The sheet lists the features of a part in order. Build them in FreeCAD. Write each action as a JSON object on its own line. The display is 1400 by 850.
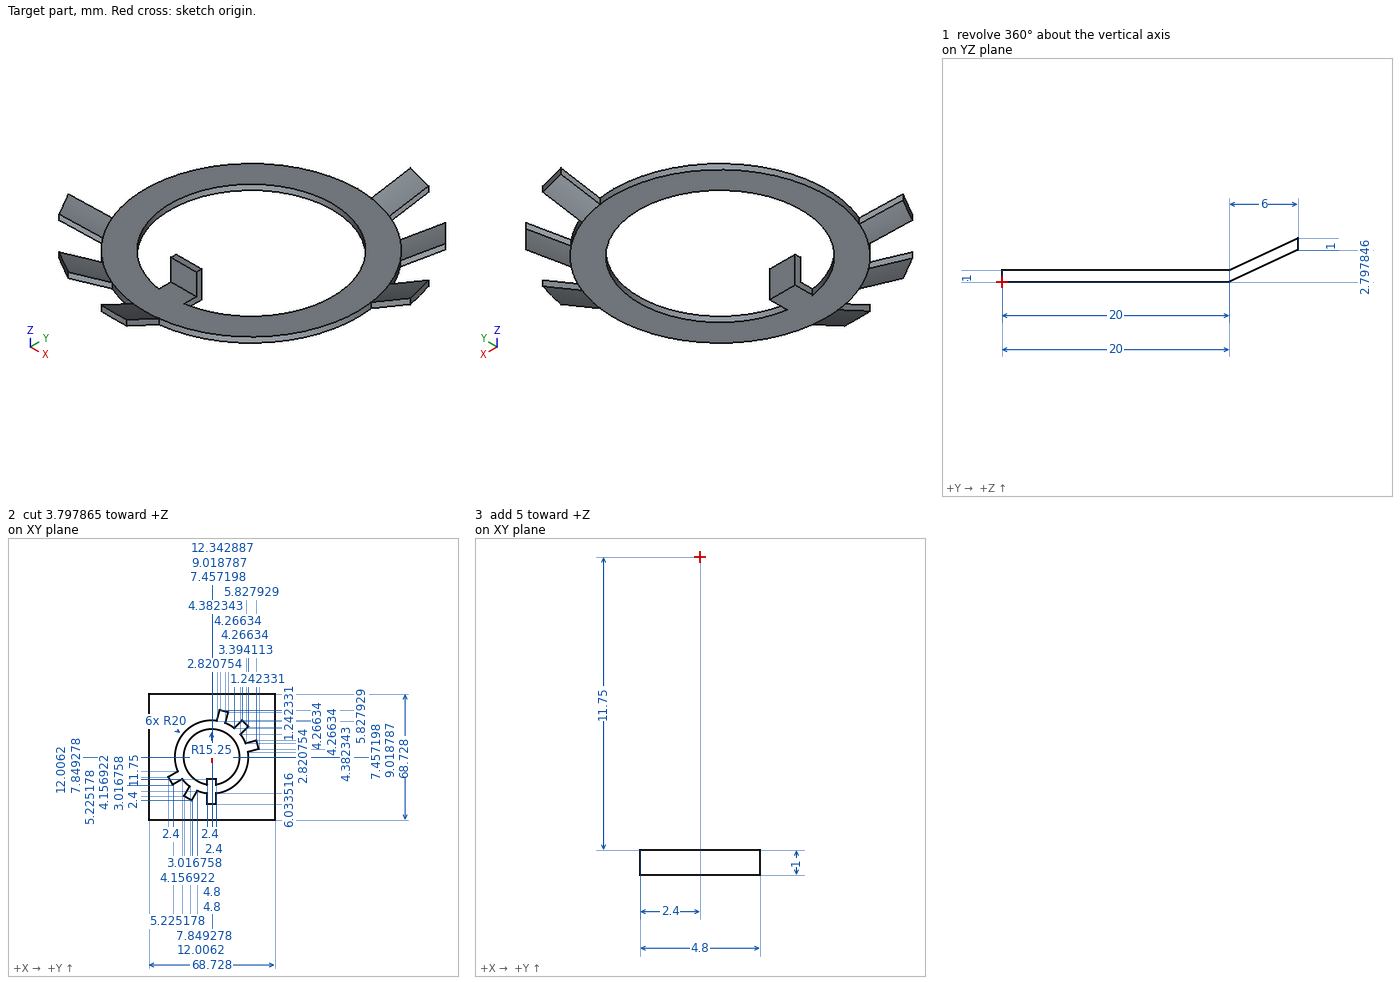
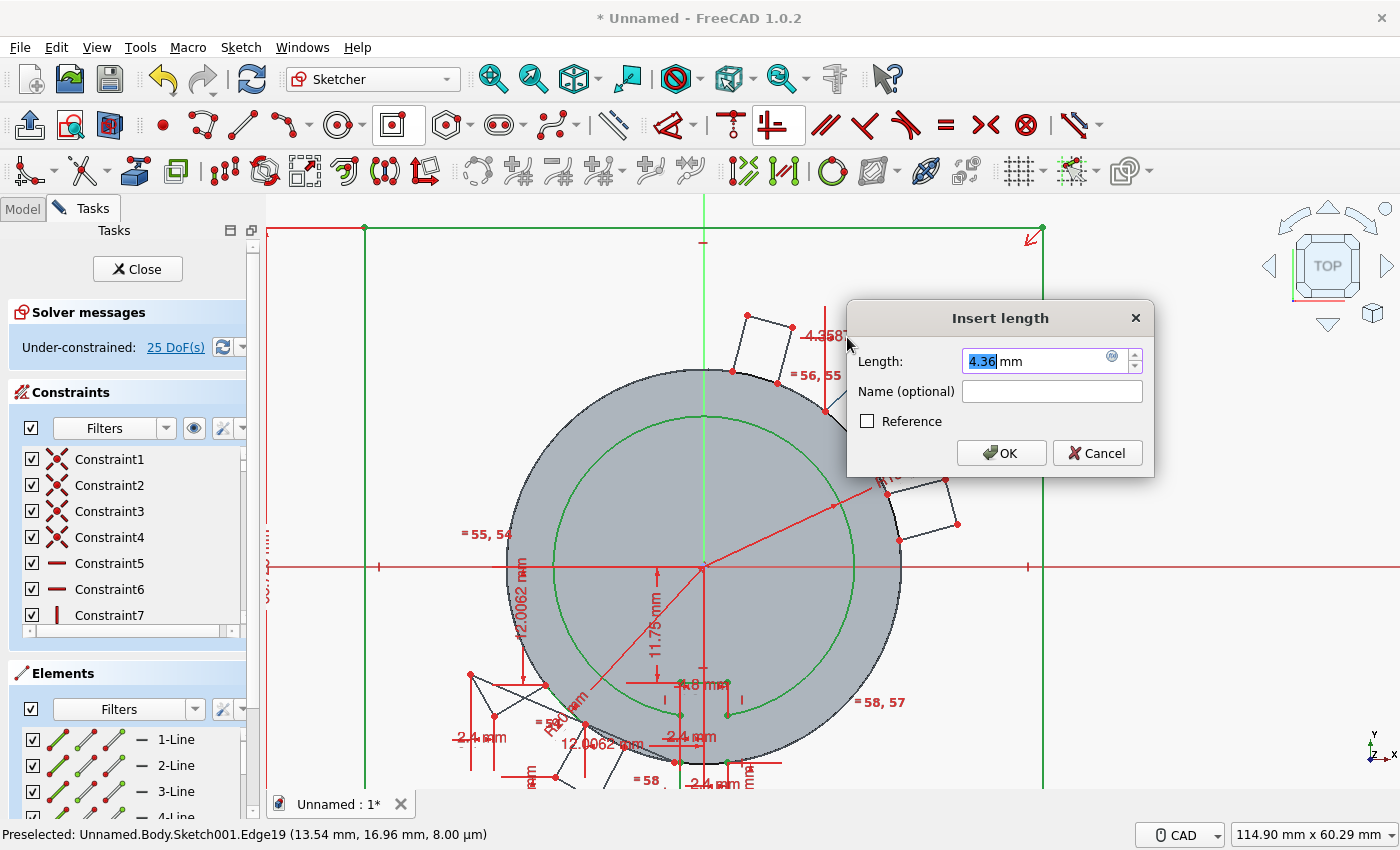
{"action": "type", "text": "4.26634"}
{"action": "key", "text": "Return"}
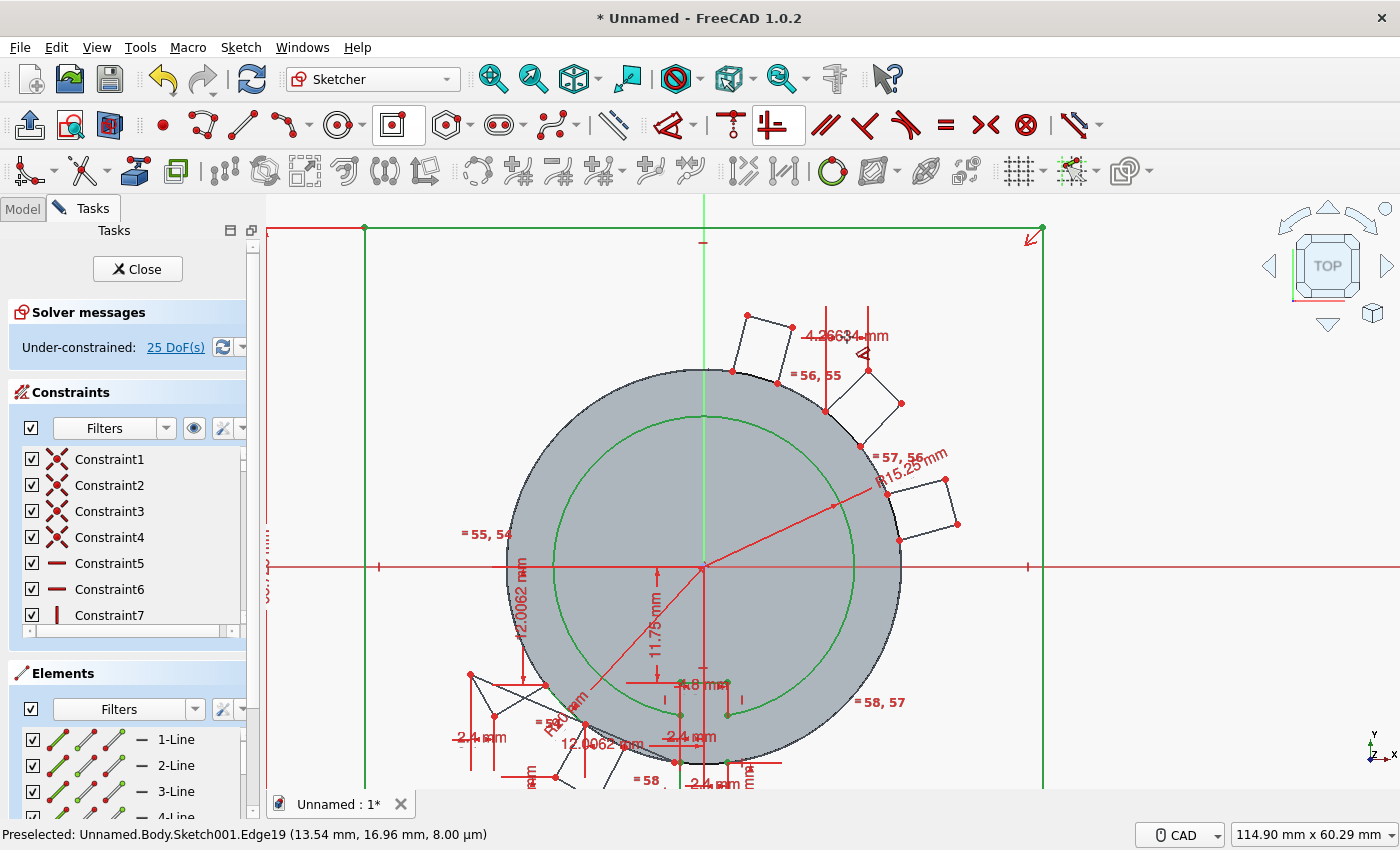
{"action": "left_click", "coordinate": [839, 399]}
{"action": "left_click", "coordinate": [902, 382]}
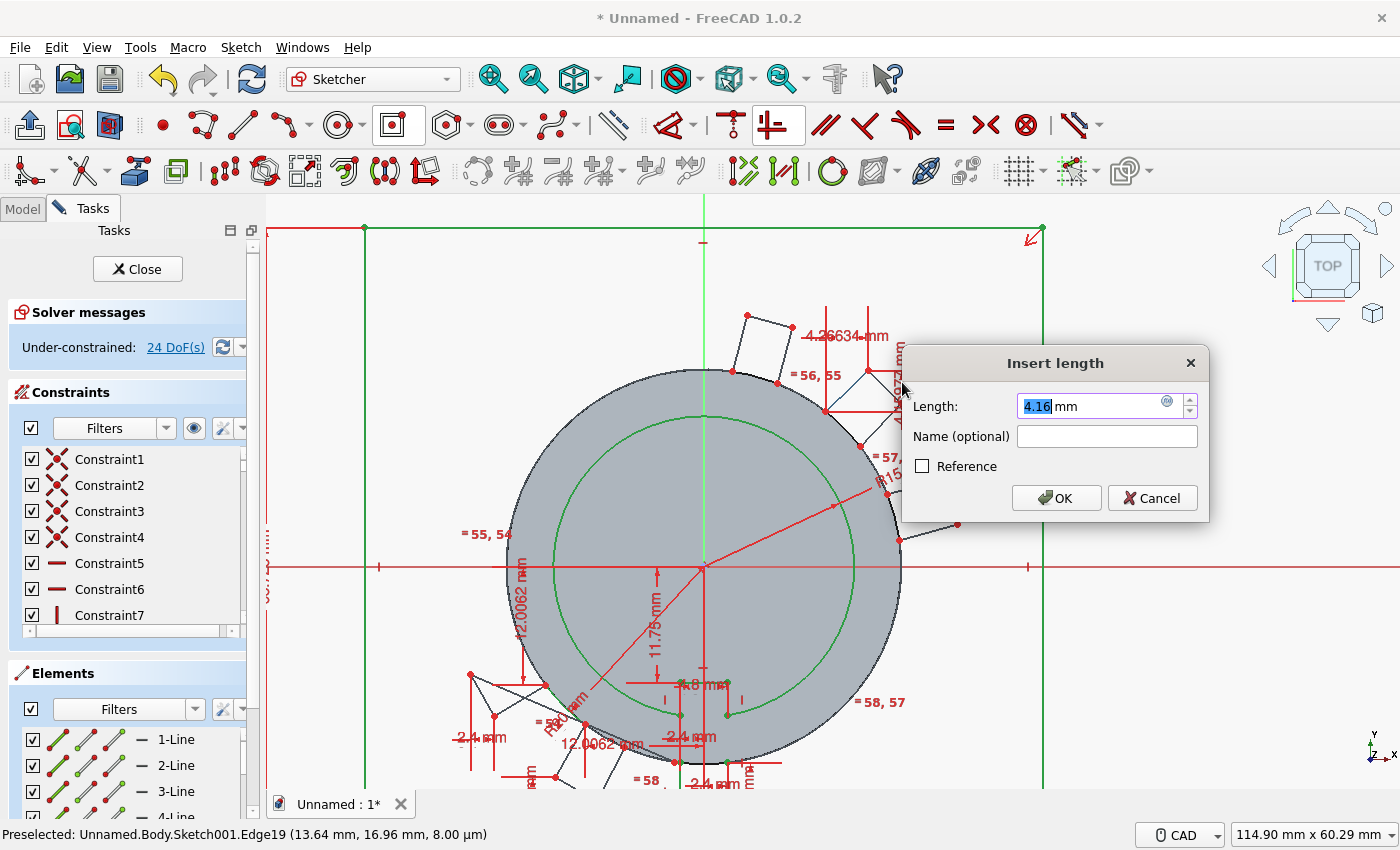
{"action": "type", "text": "4.26634"}
{"action": "key", "text": "Return"}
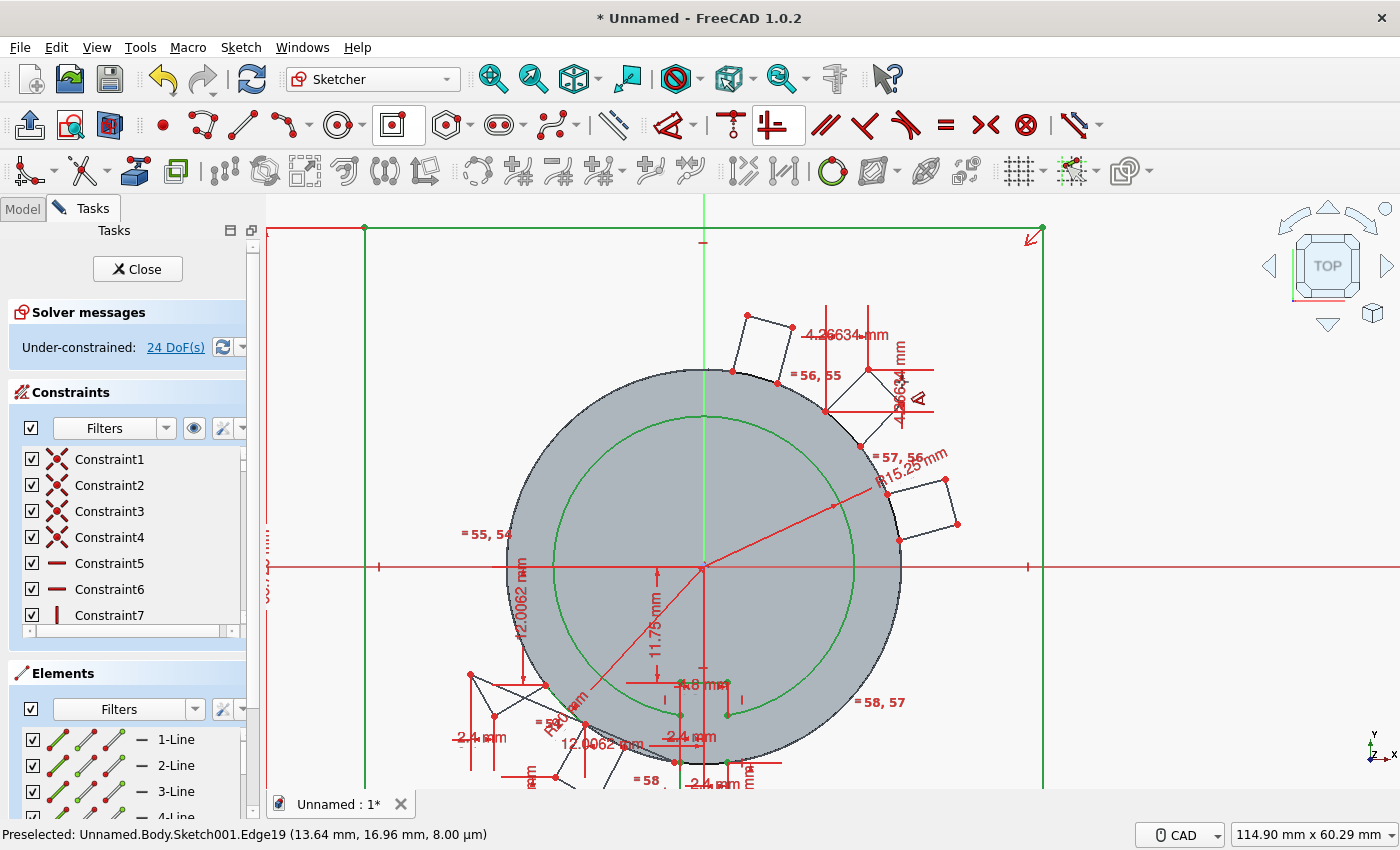
{"action": "left_click", "coordinate": [889, 417]}
{"action": "left_click", "coordinate": [871, 505]}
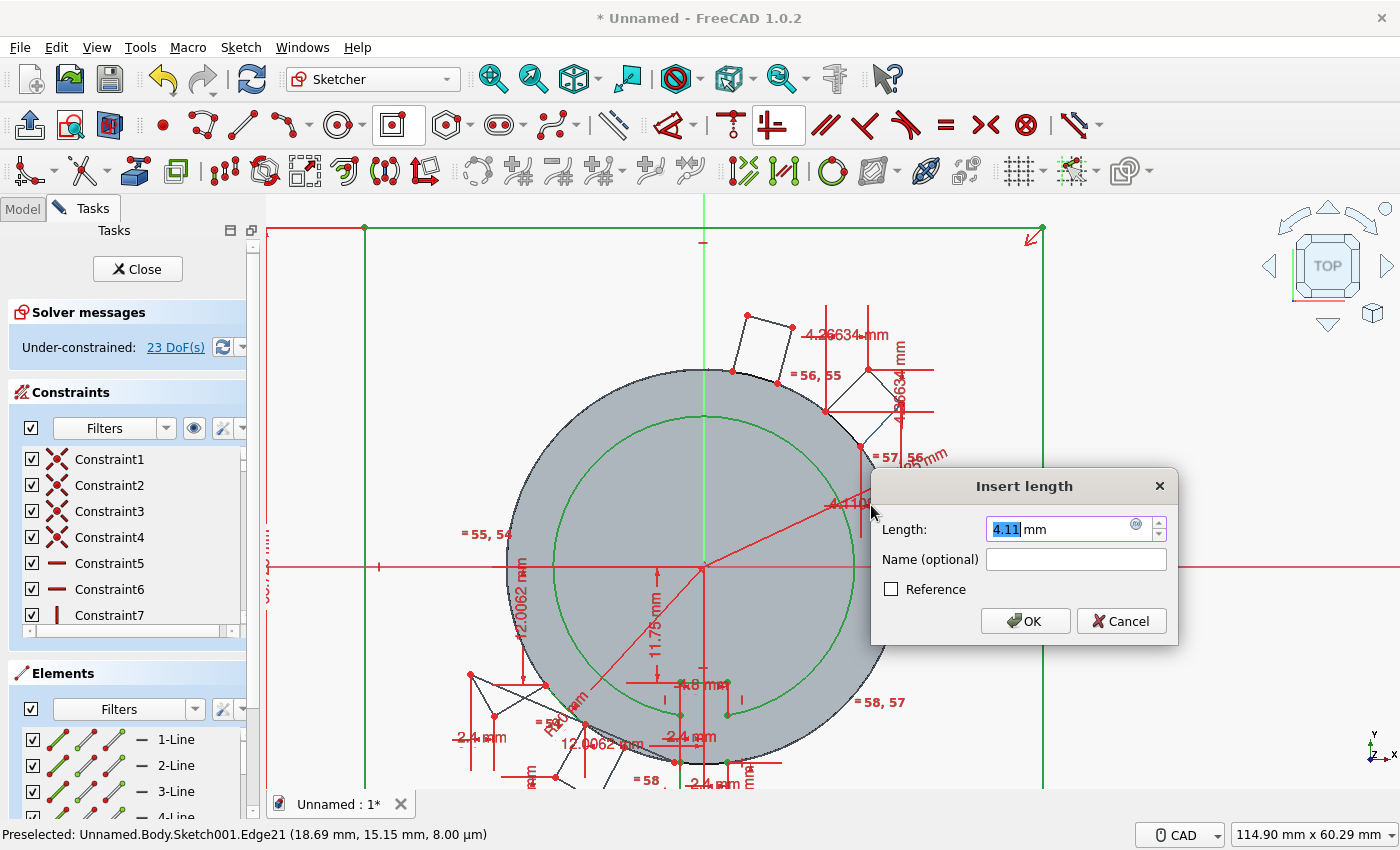
{"action": "type", "text": "4.26634"}
{"action": "key", "text": "Return"}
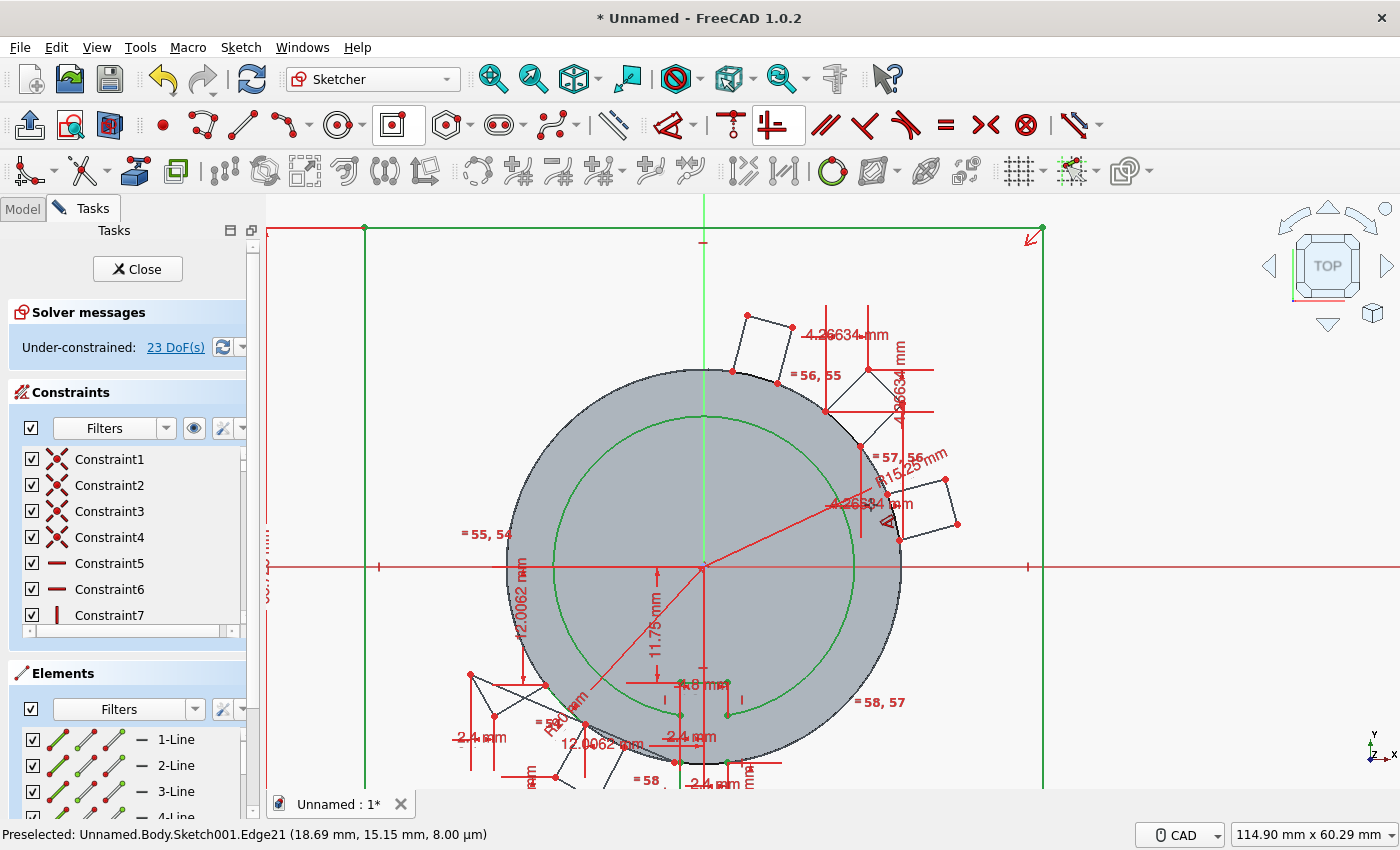
{"action": "left_click", "coordinate": [890, 417]}
{"action": "left_click", "coordinate": [937, 425]}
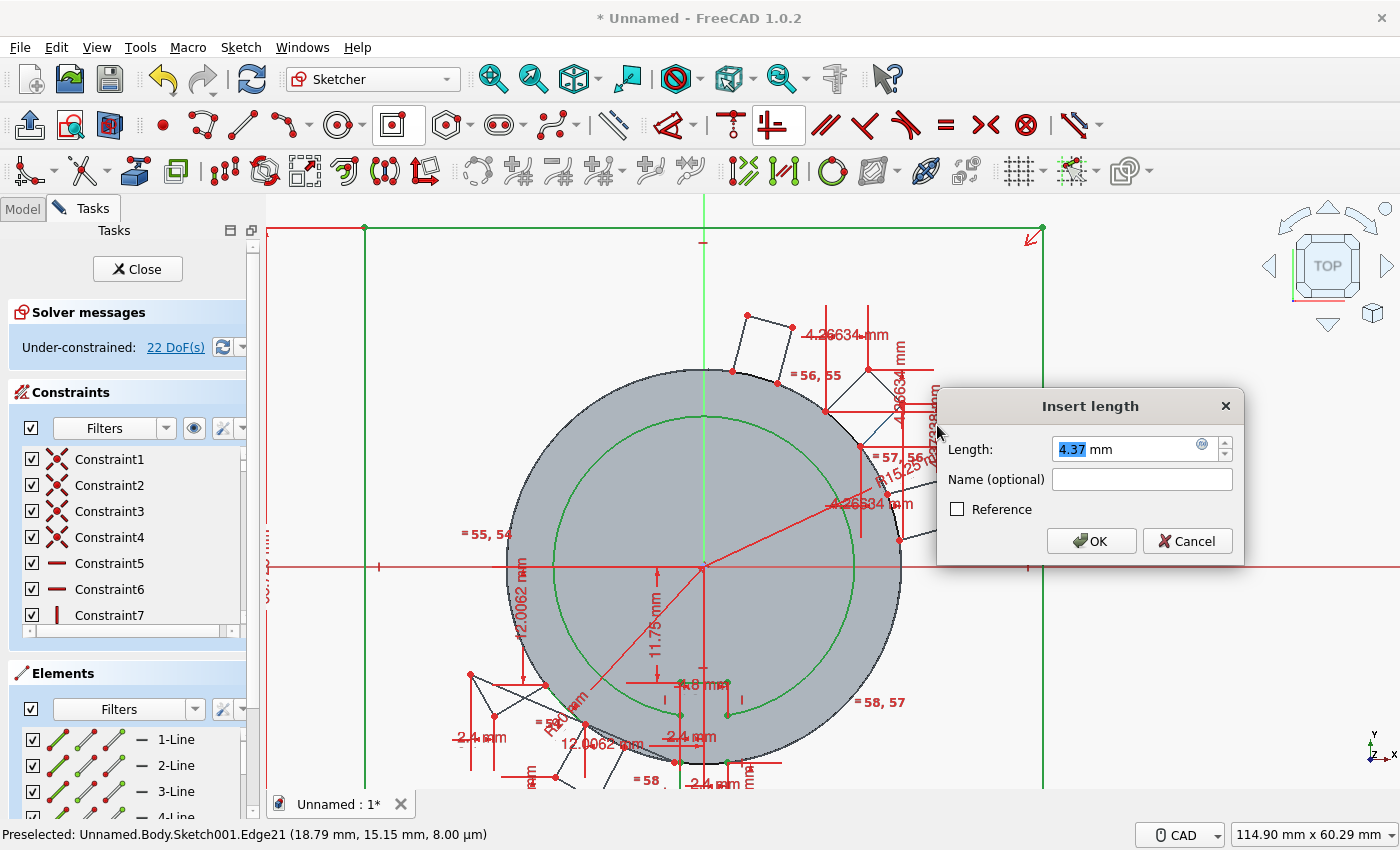
{"action": "type", "text": "4.26634"}
{"action": "key", "text": "Return"}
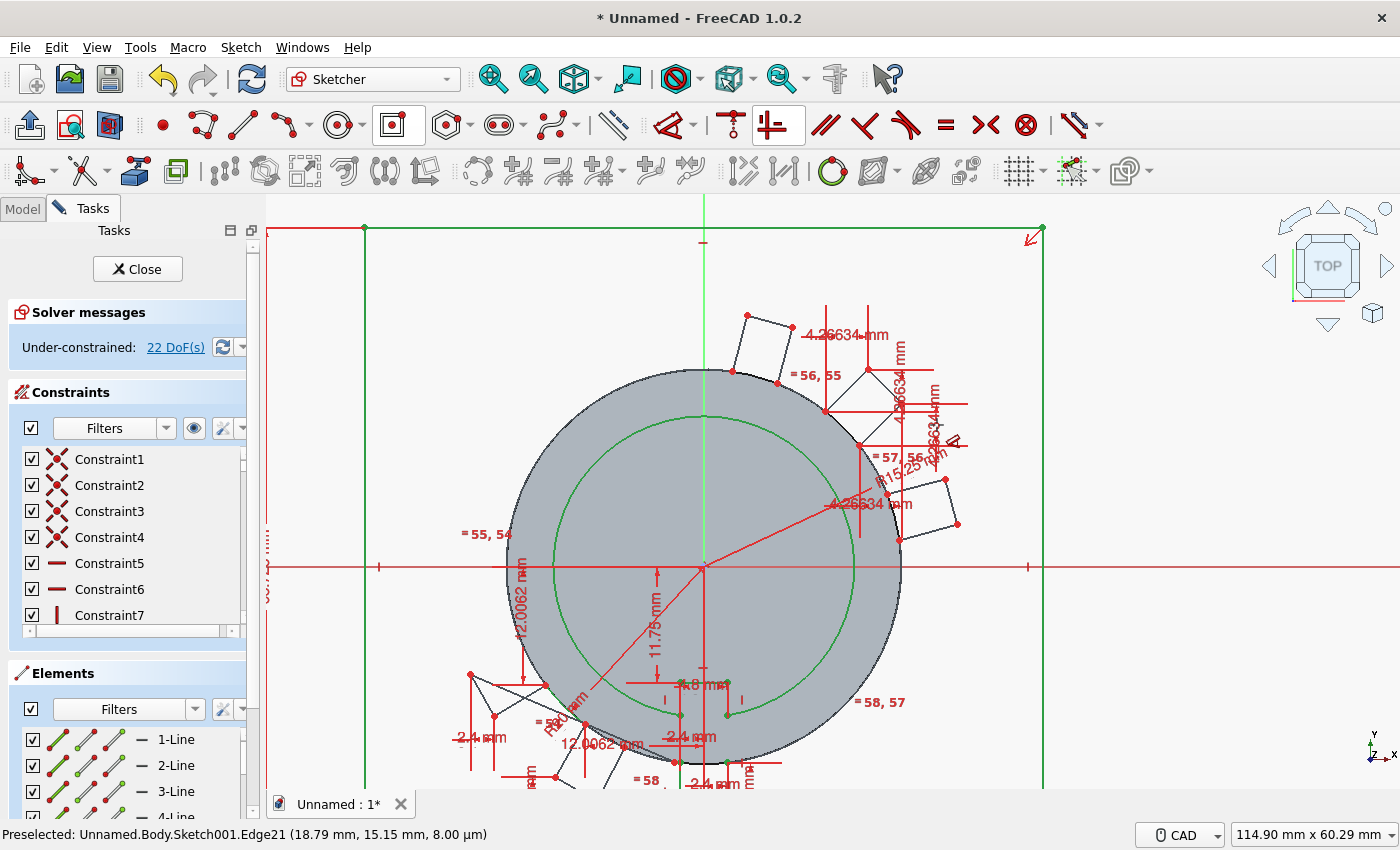
{"action": "left_click", "coordinate": [625, 748]}
{"action": "left_click", "coordinate": [664, 533]}